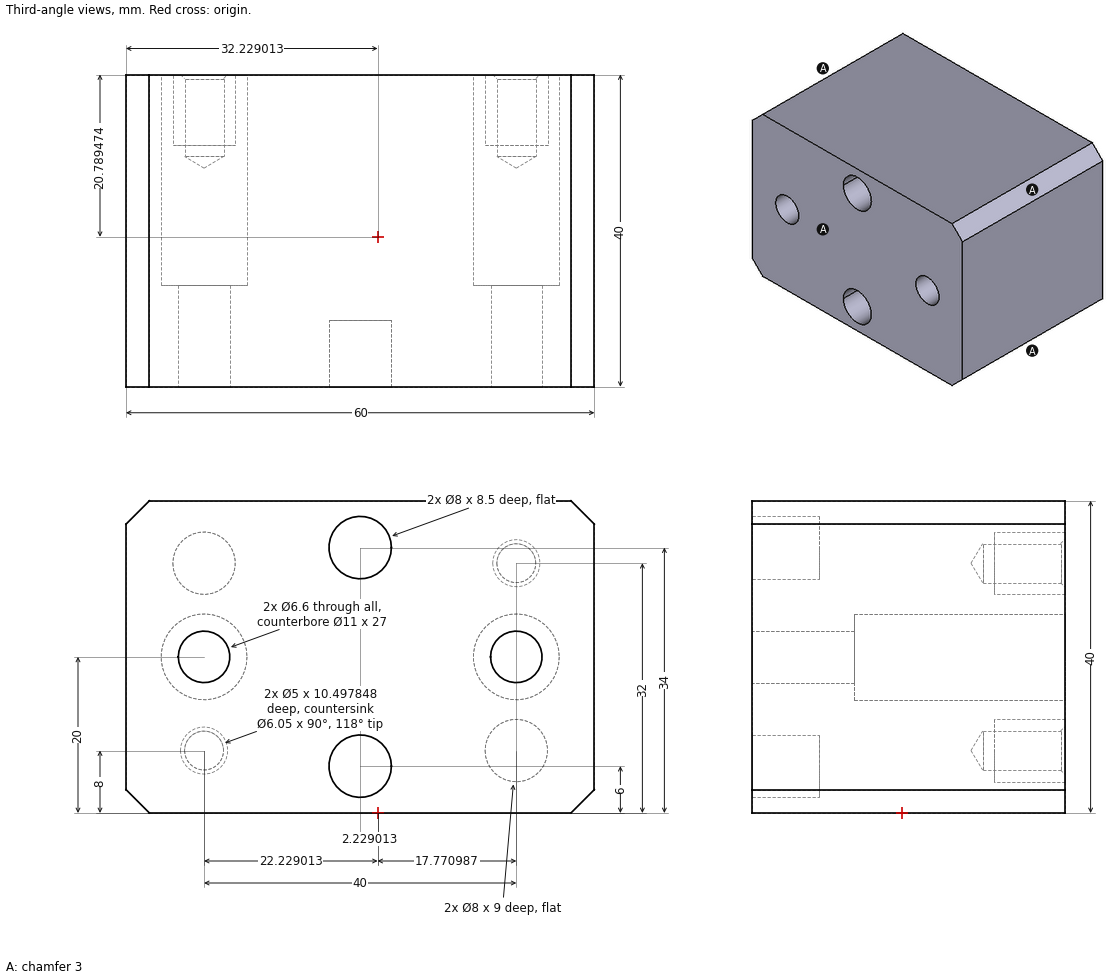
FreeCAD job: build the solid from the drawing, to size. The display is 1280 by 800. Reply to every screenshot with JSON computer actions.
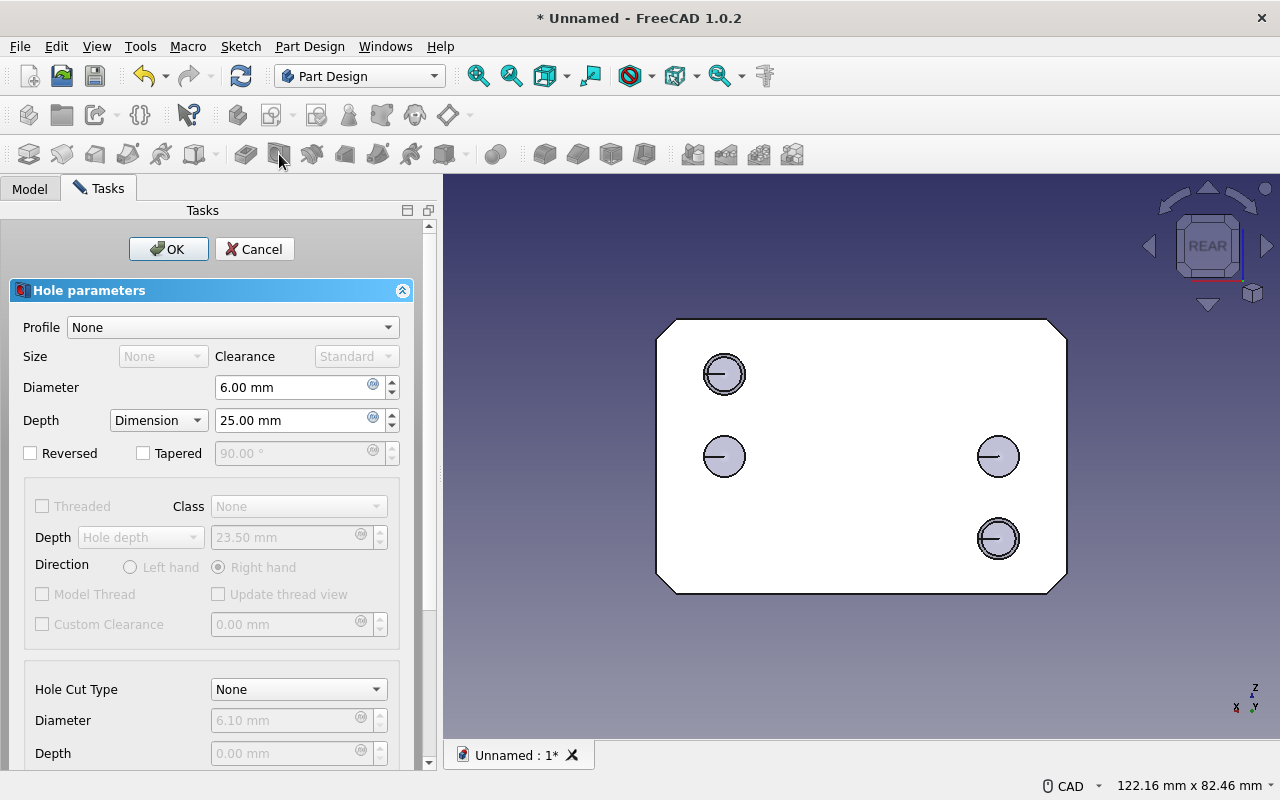
{"action": "triple_click", "coordinate": [300, 388]}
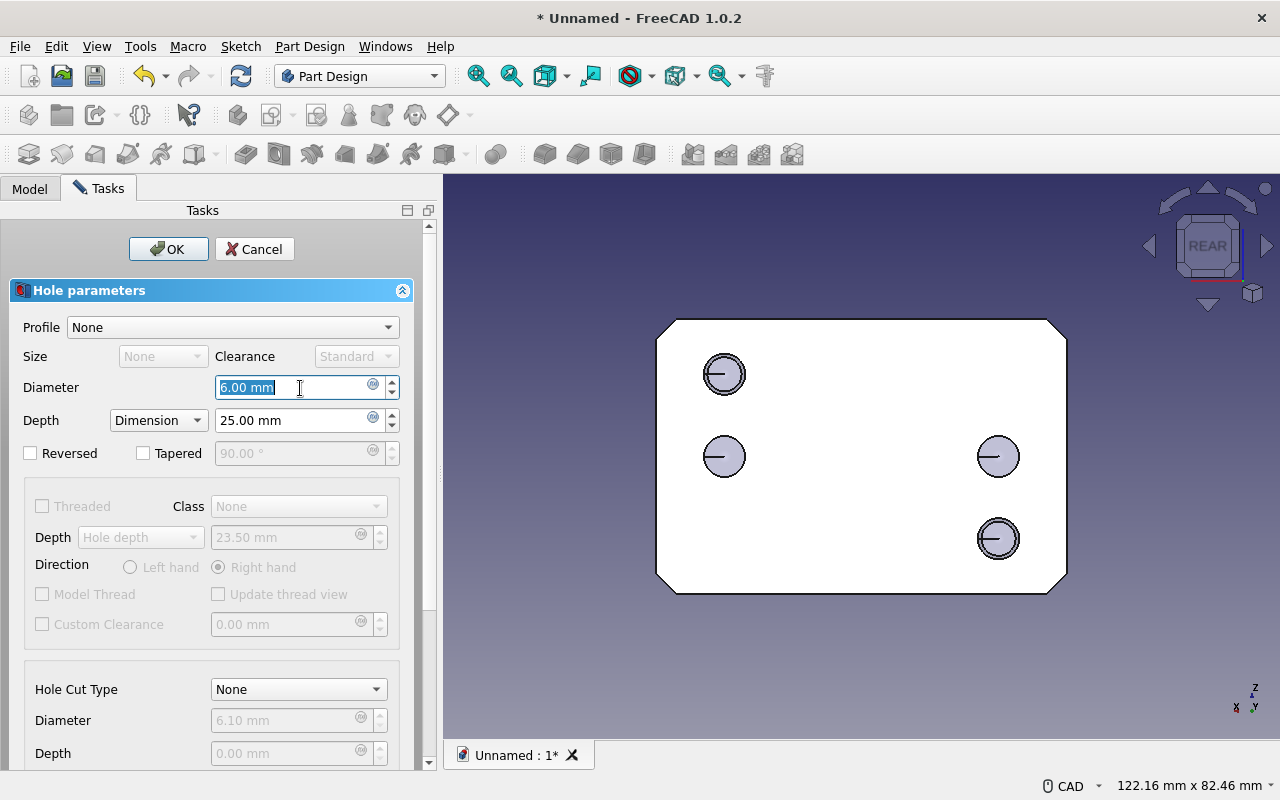
{"action": "type", "text": "6.6"}
{"action": "key", "text": "Tab"}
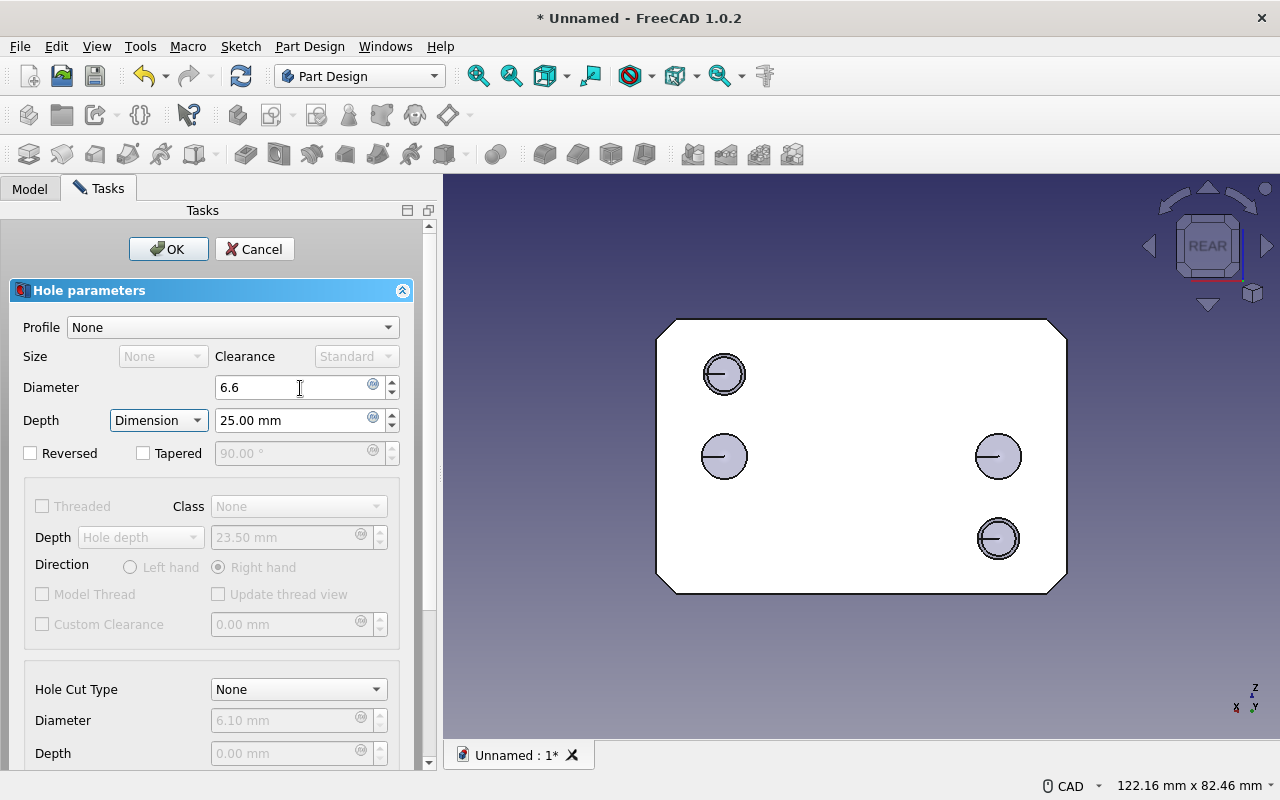
{"action": "left_click", "coordinate": [160, 420]}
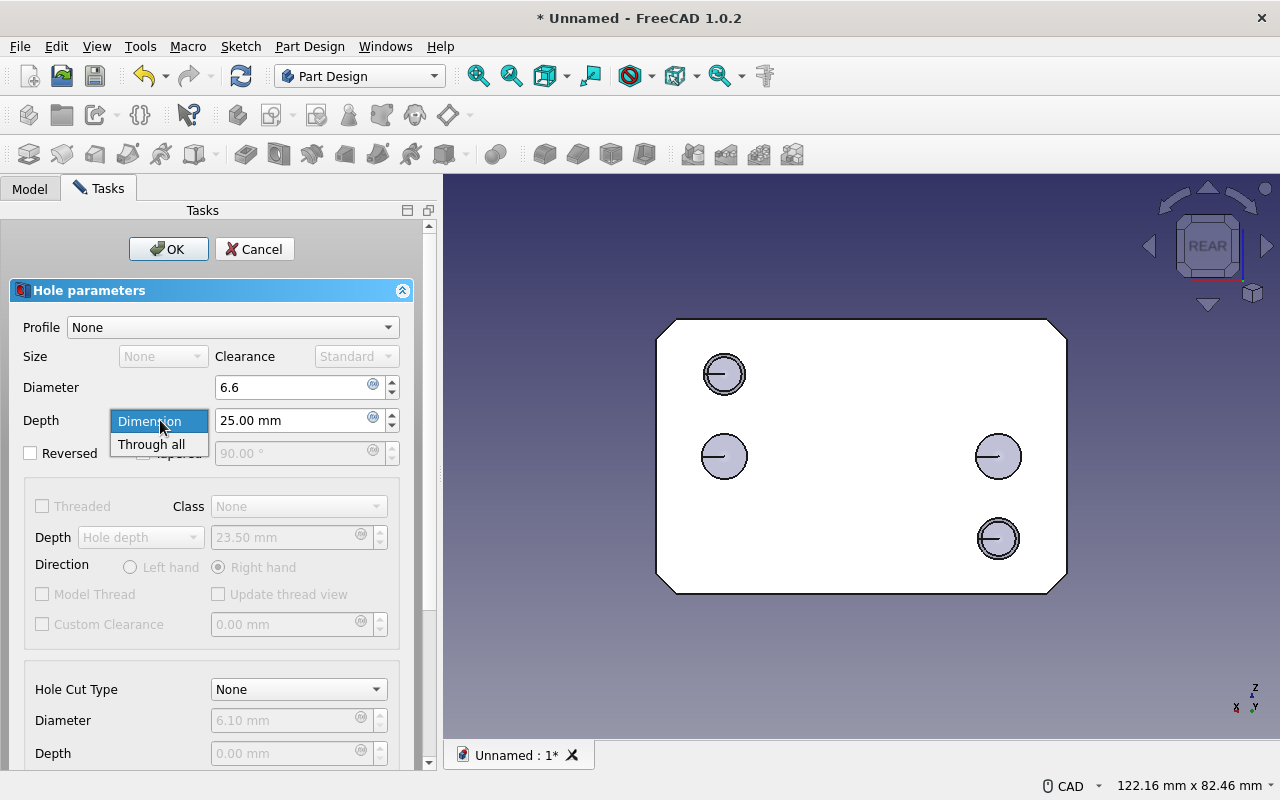
{"action": "left_click", "coordinate": [158, 444]}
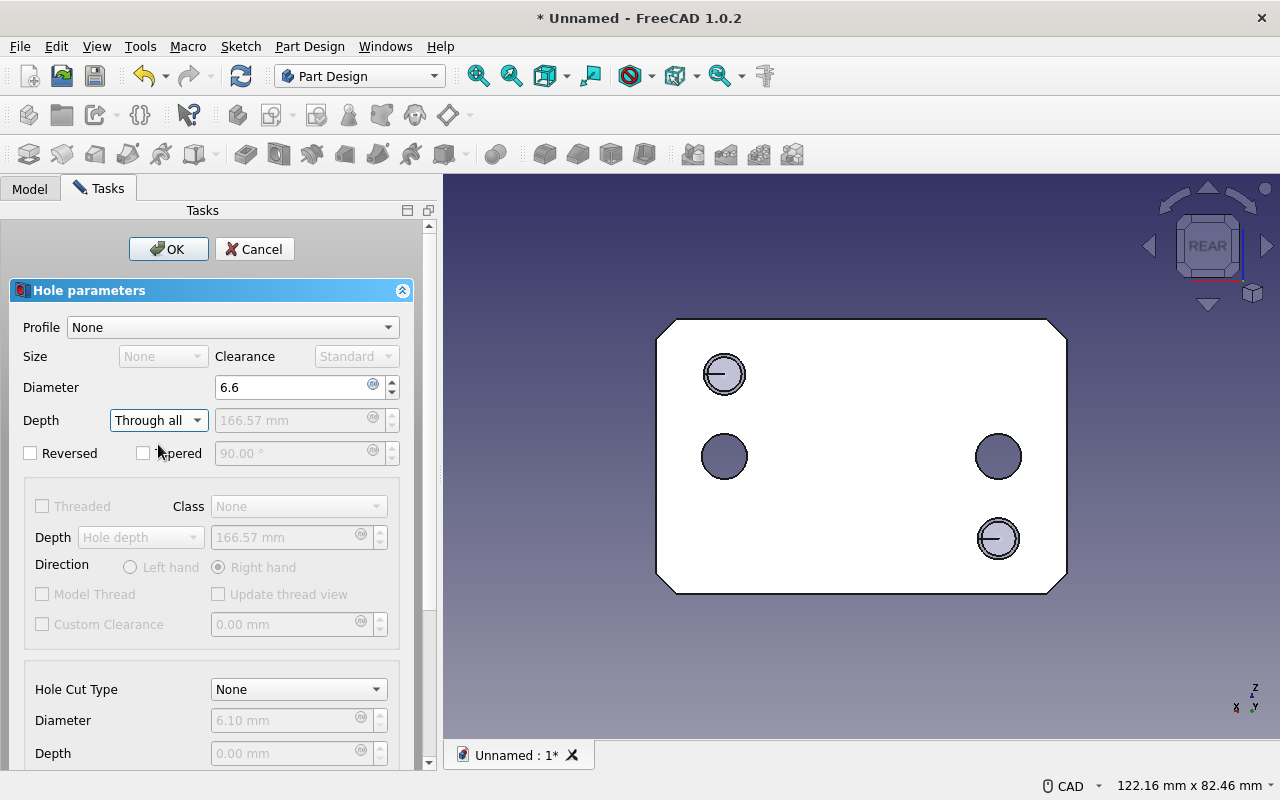
{"action": "left_click", "coordinate": [300, 690]}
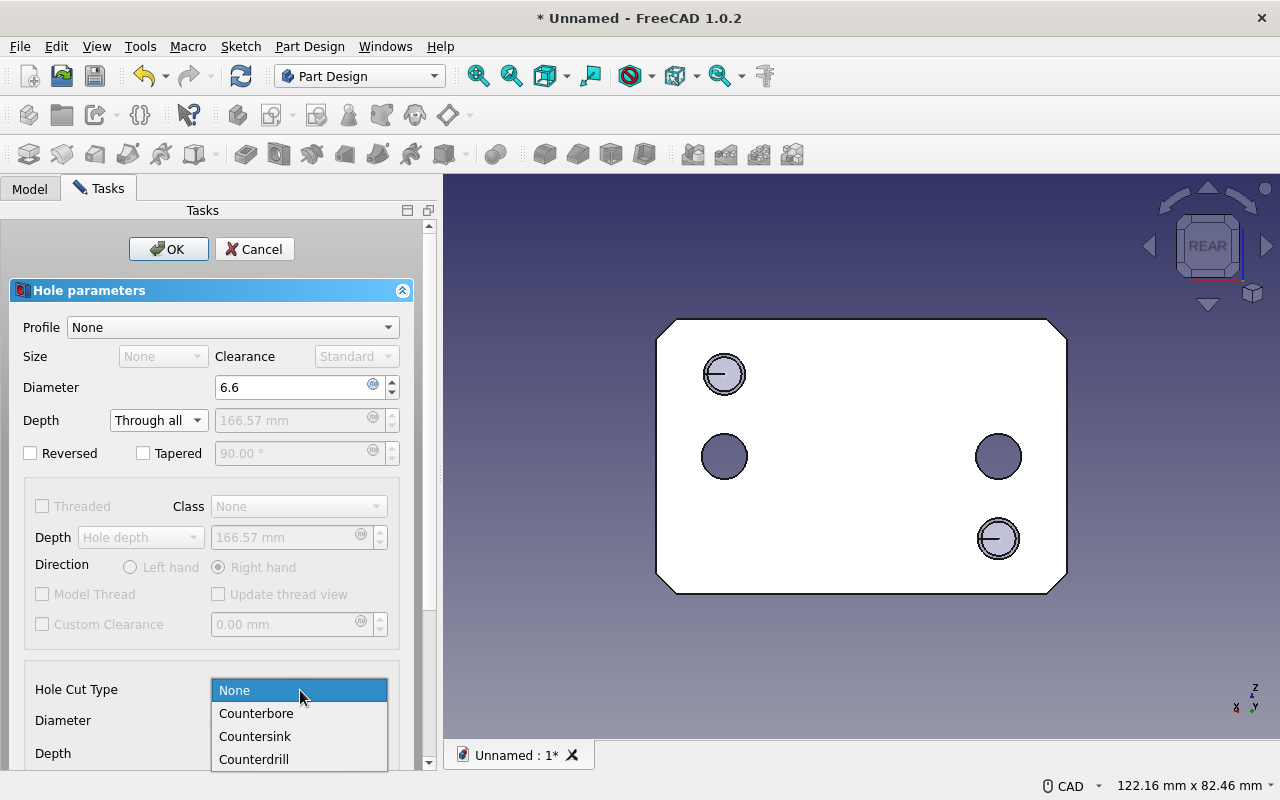
{"action": "left_click", "coordinate": [298, 714]}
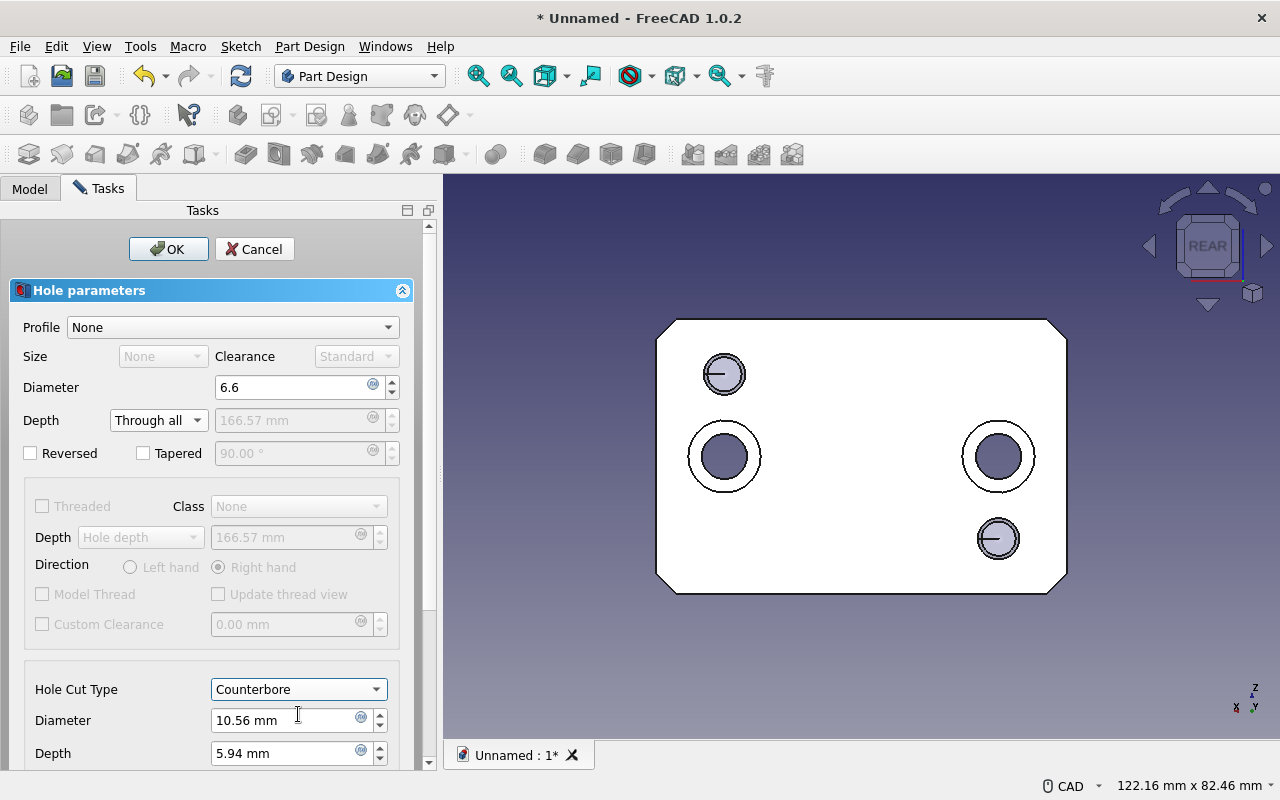
{"action": "triple_click", "coordinate": [292, 720]}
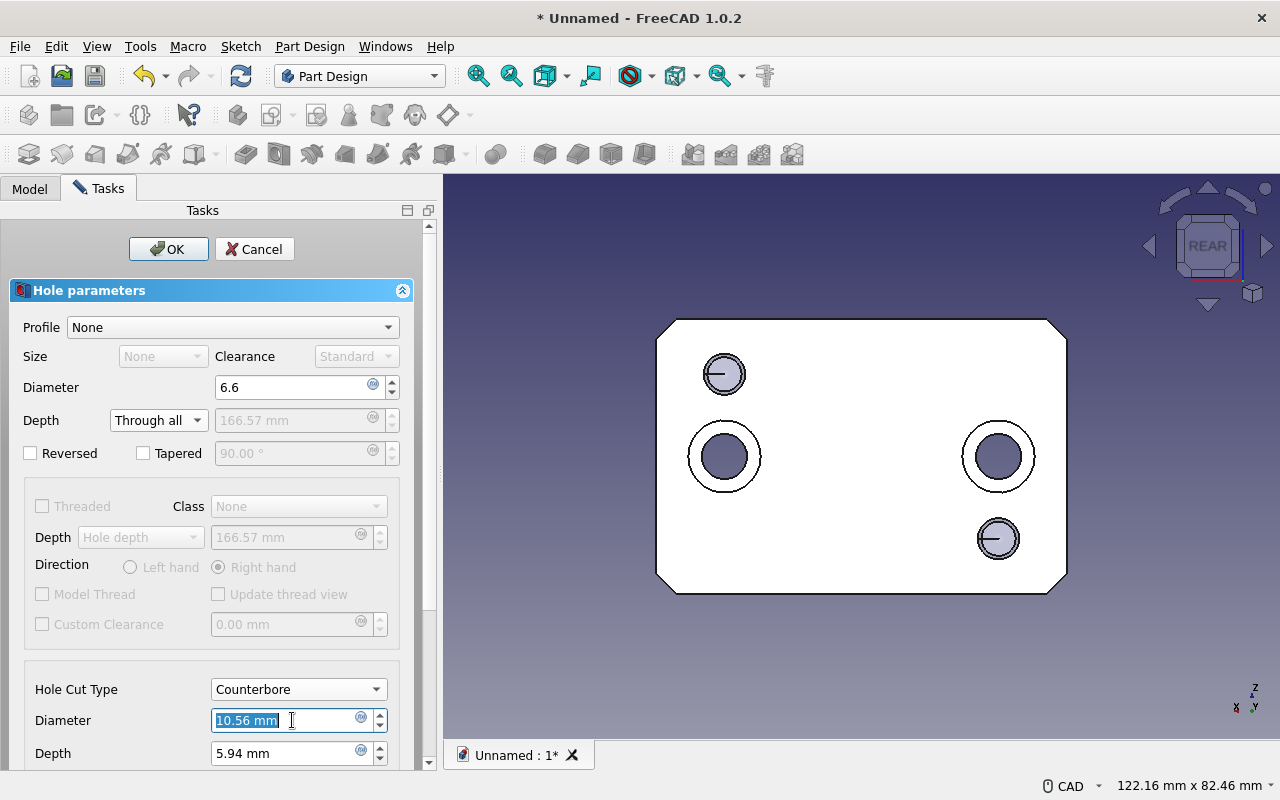
{"action": "type", "text": "11"}
{"action": "key", "text": "Tab"}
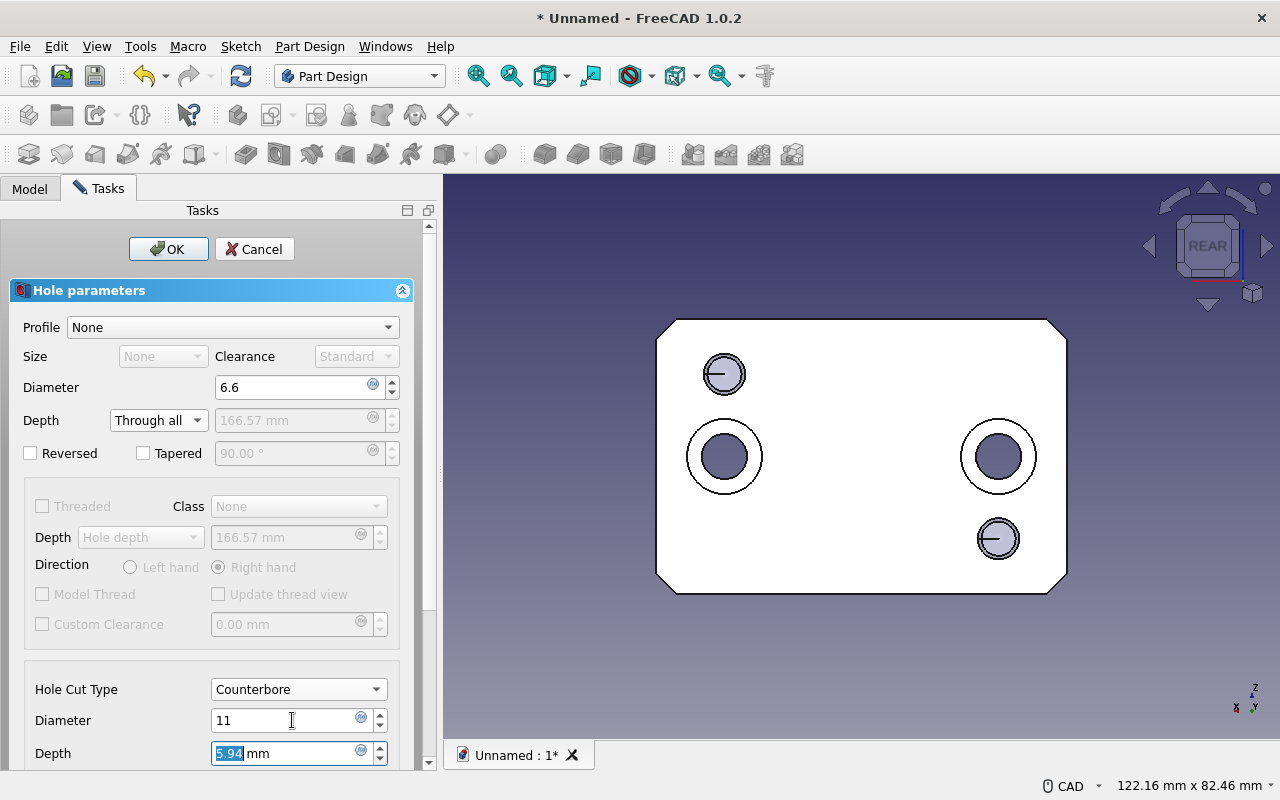
{"action": "type", "text": "27"}
{"action": "key", "text": "Tab"}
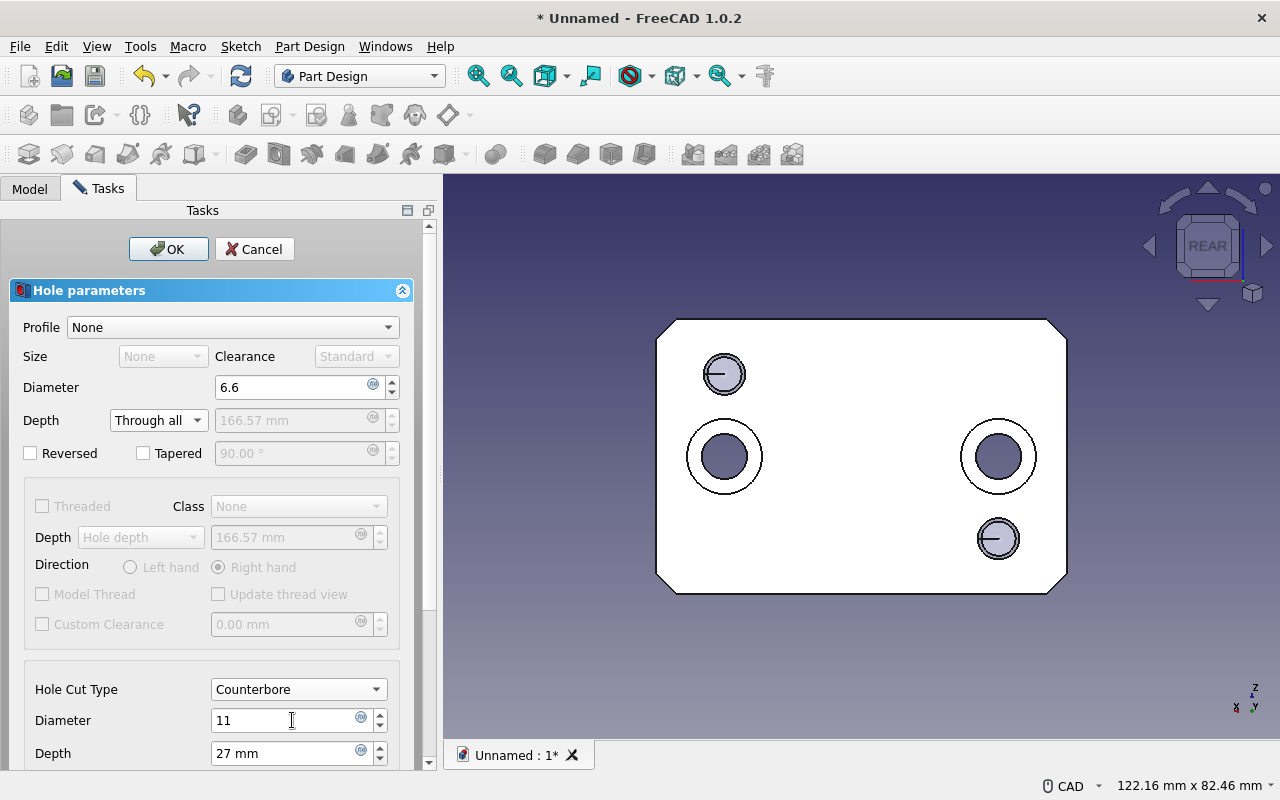
{"action": "left_click", "coordinate": [169, 249]}